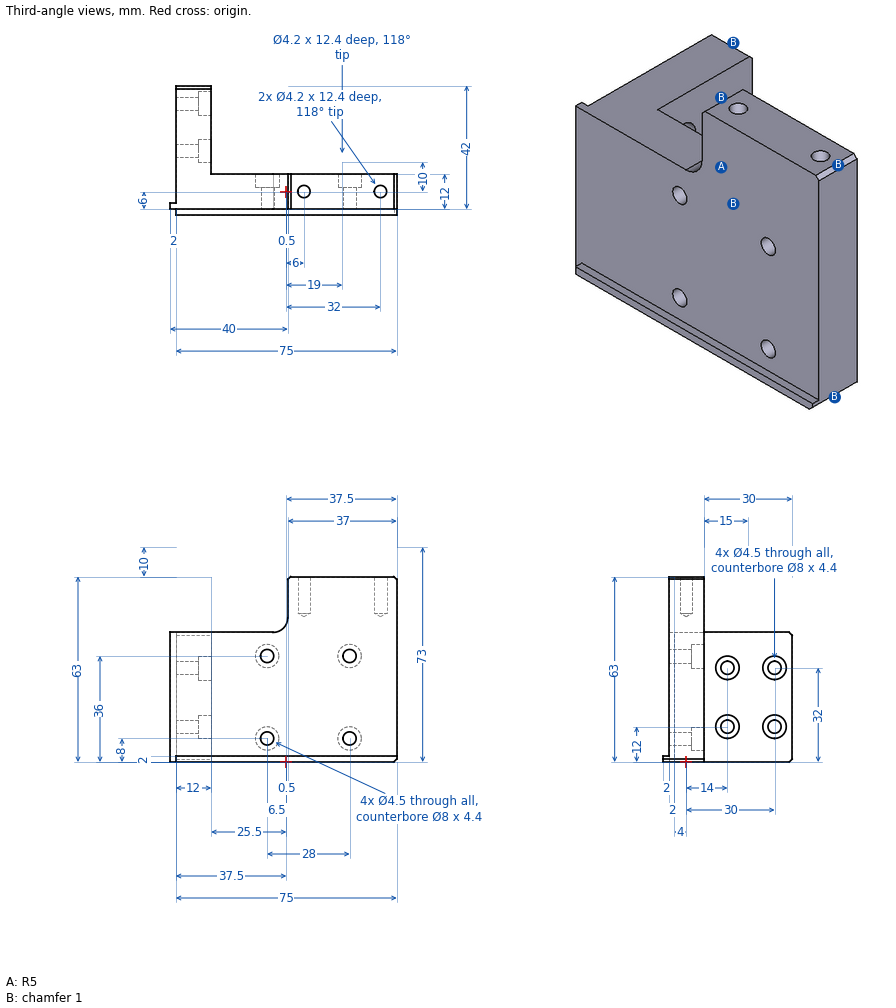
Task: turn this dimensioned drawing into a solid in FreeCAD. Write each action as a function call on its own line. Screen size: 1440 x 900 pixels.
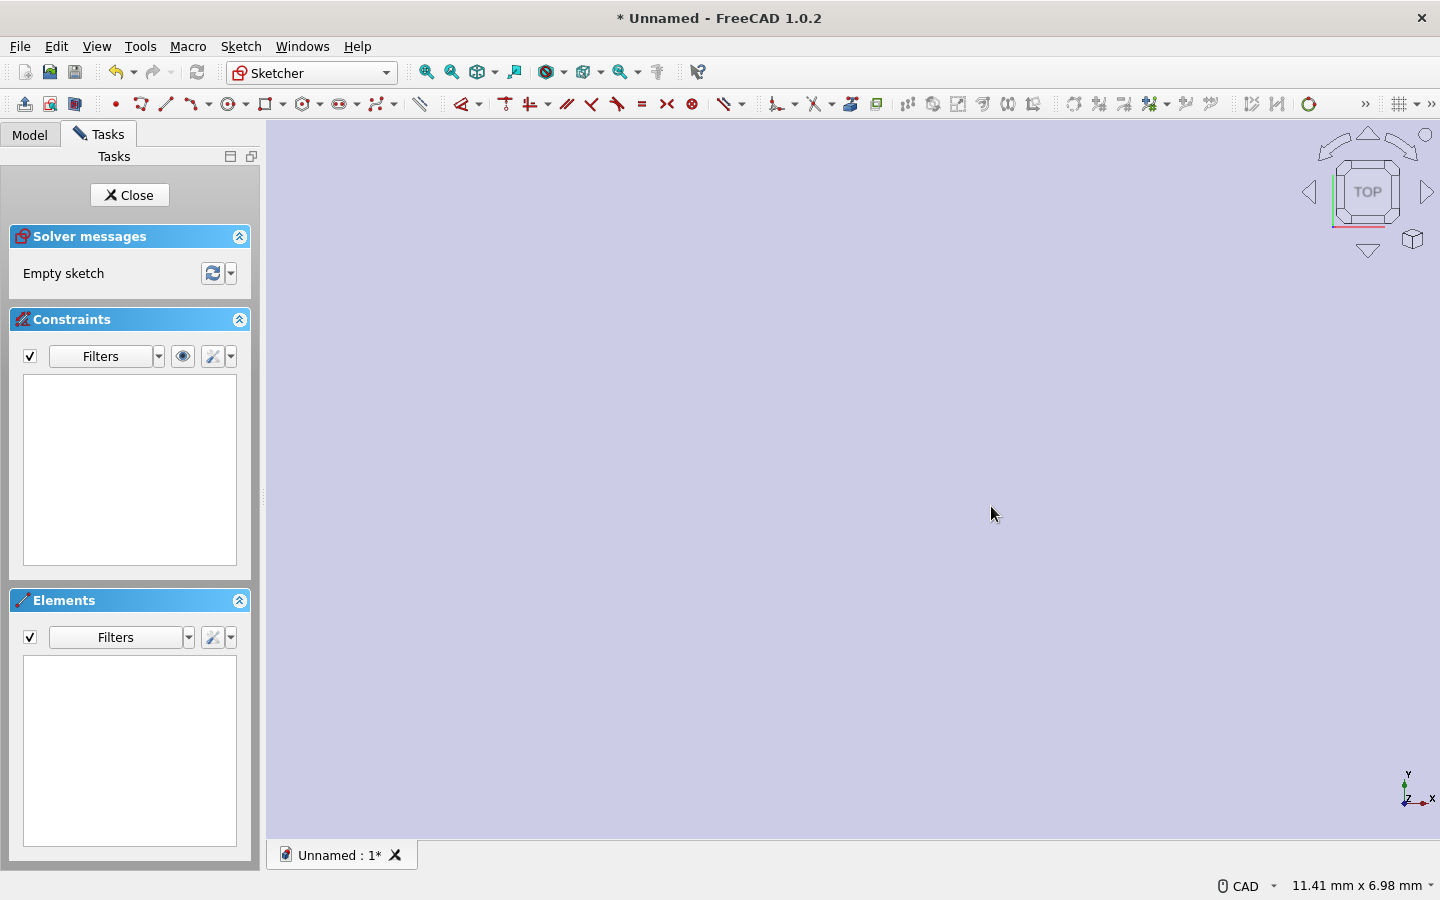
key(g)
key(c)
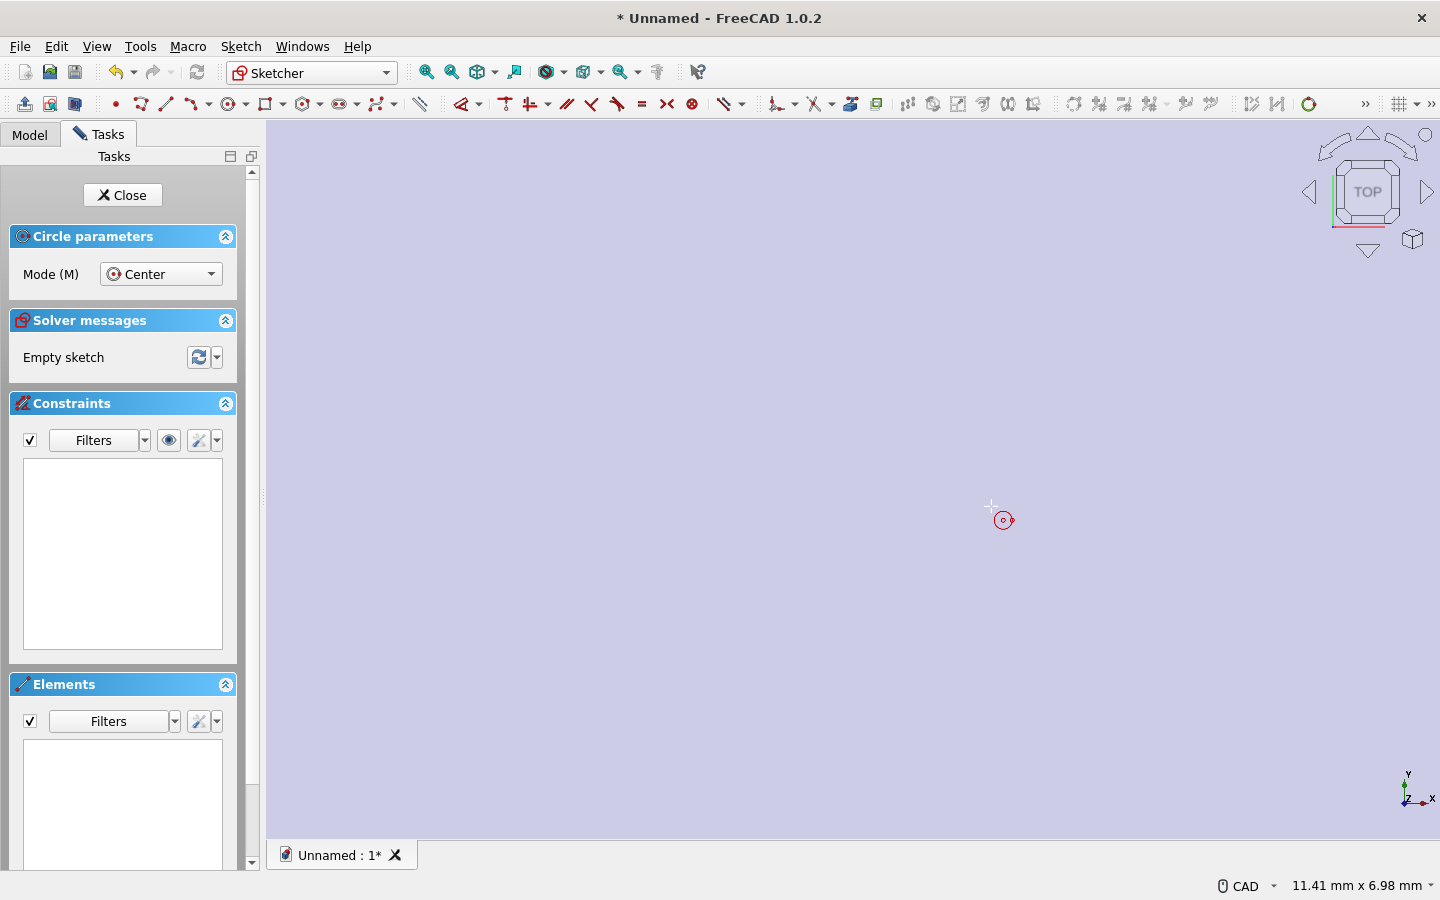
click(771, 474)
move(924, 321)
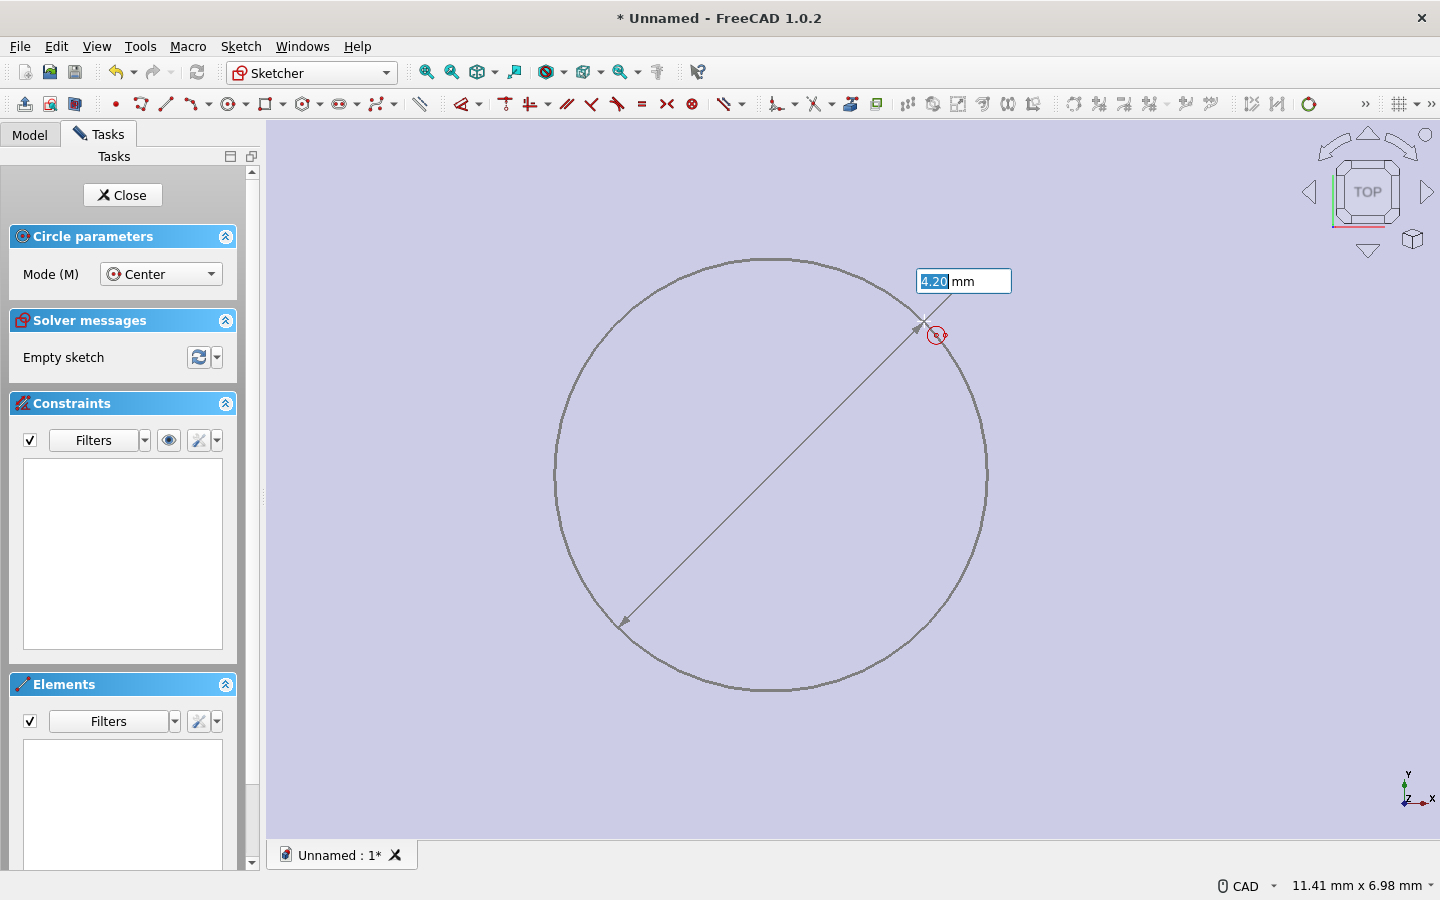
text(4.2)
key(Return)
key(Escape)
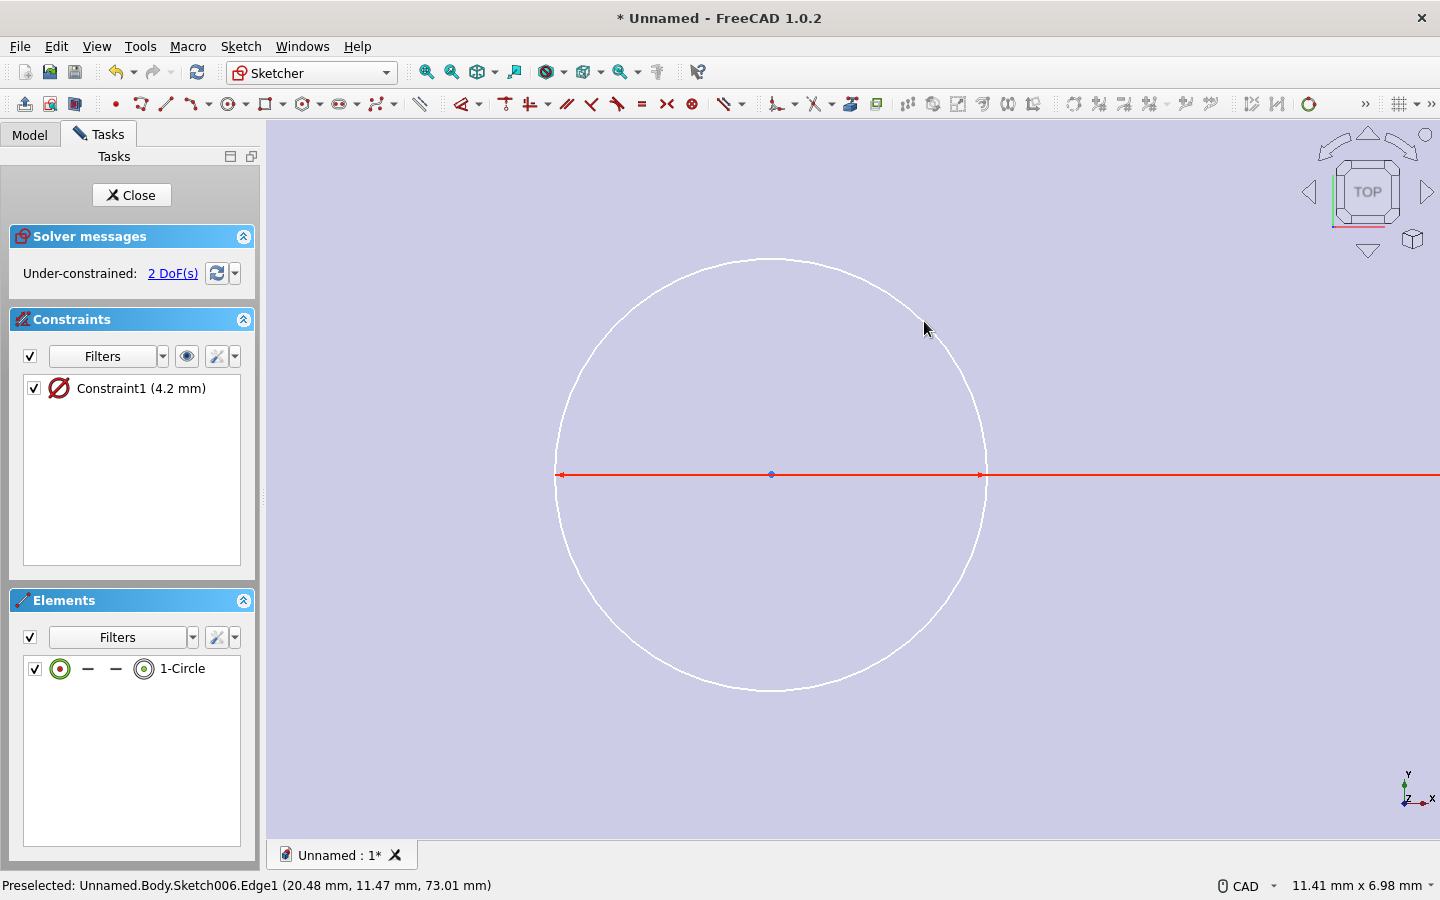
key(d)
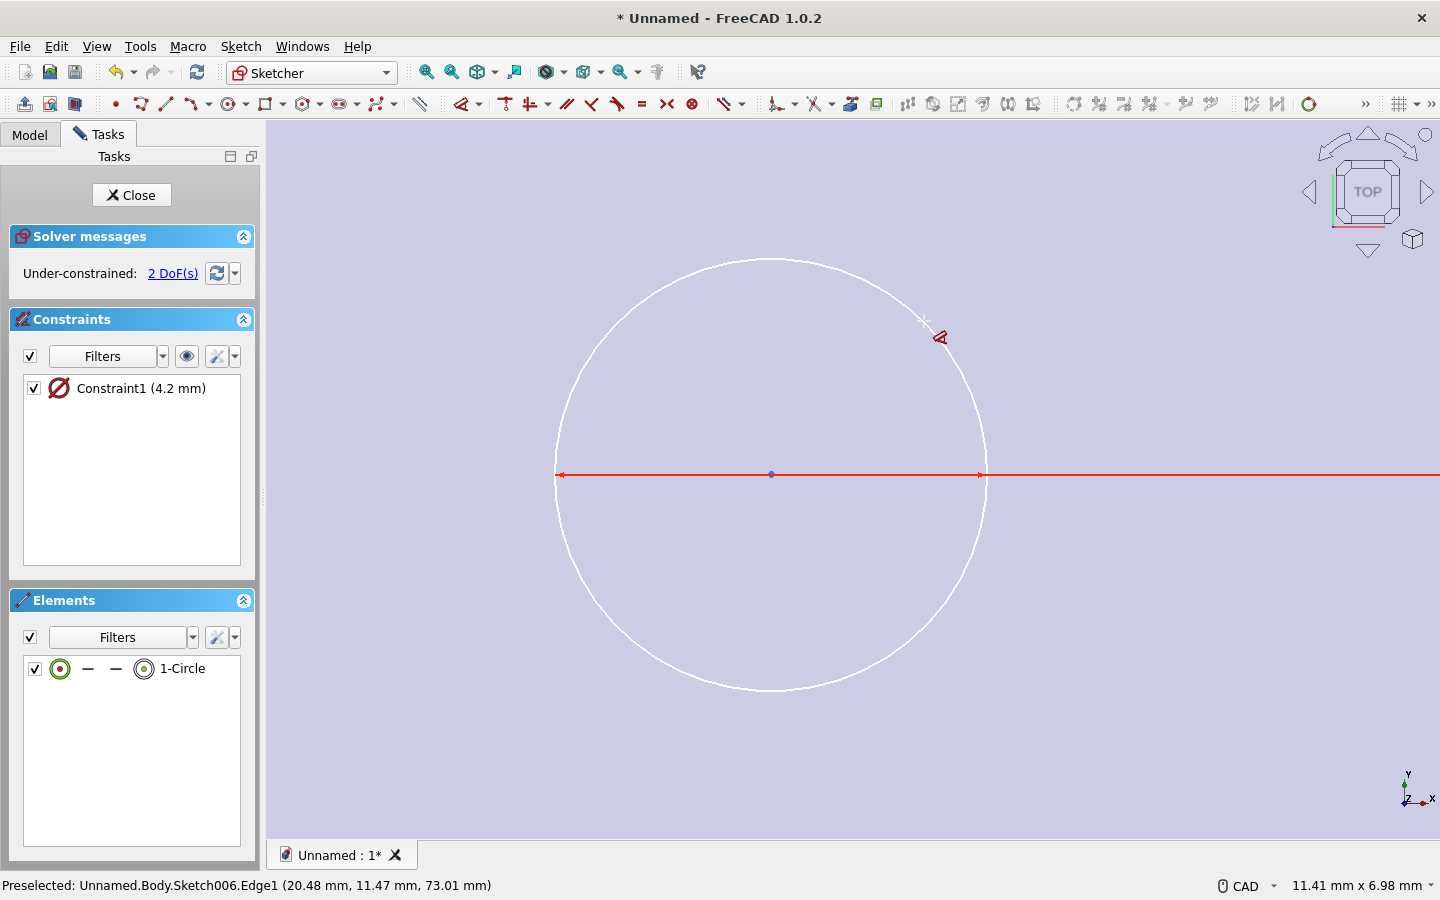
click(771, 475)
click(533, 441)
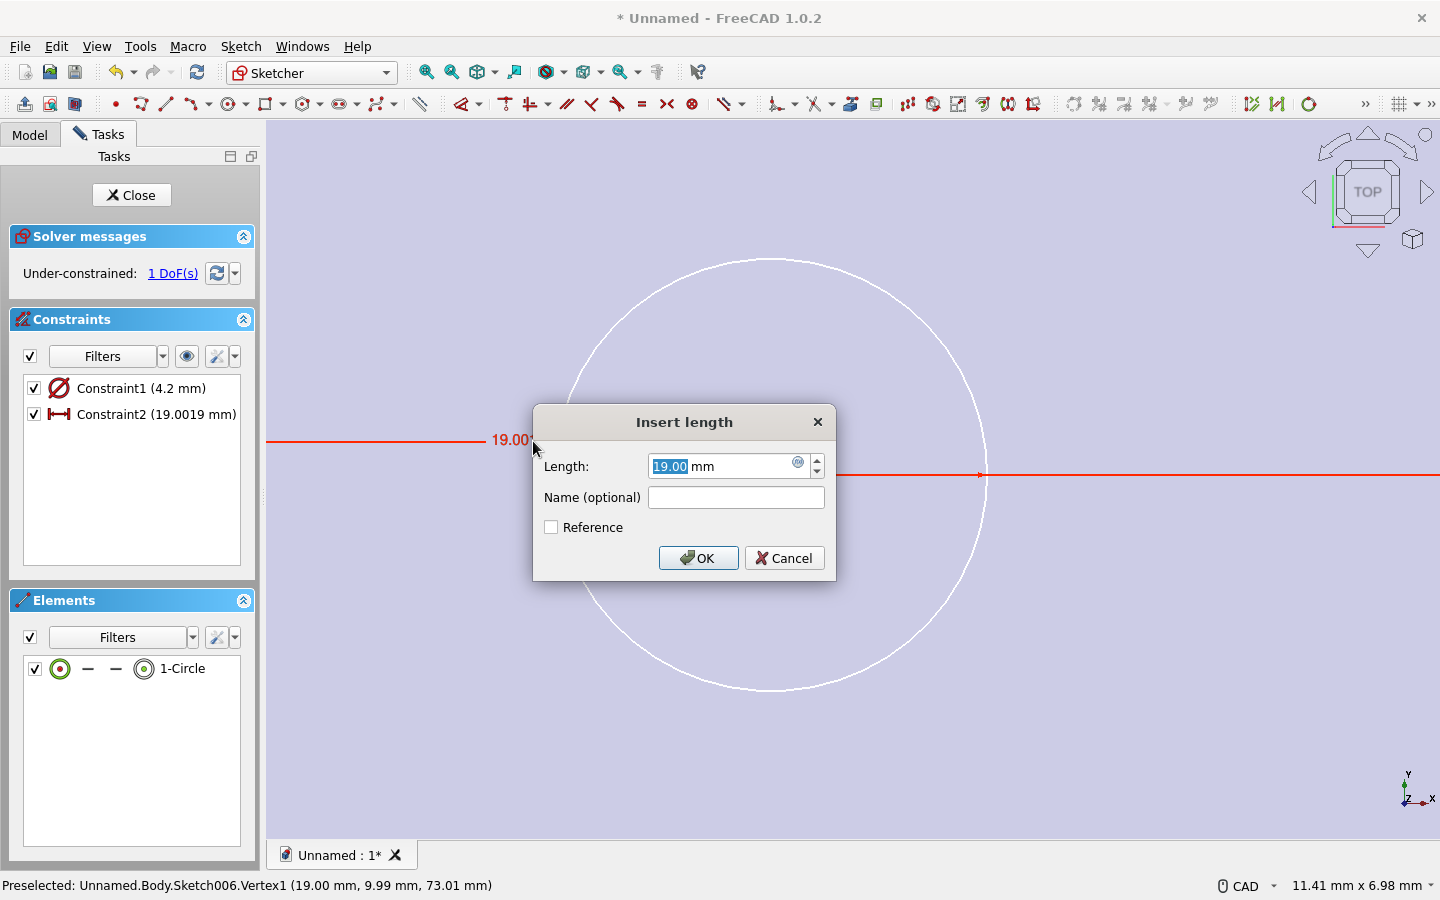
text(19)
key(Return)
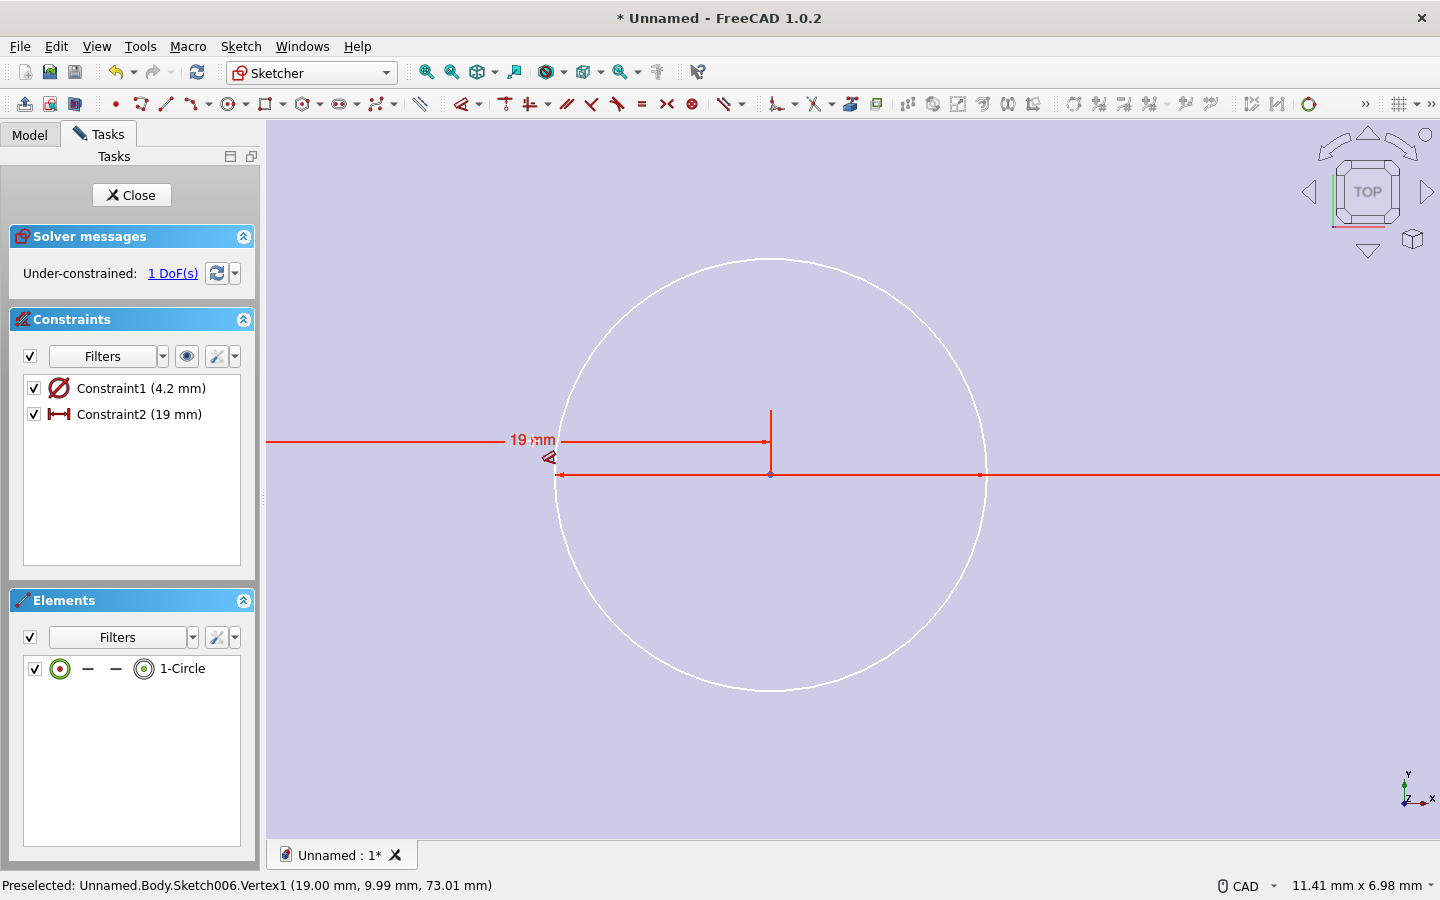
click(771, 475)
click(805, 643)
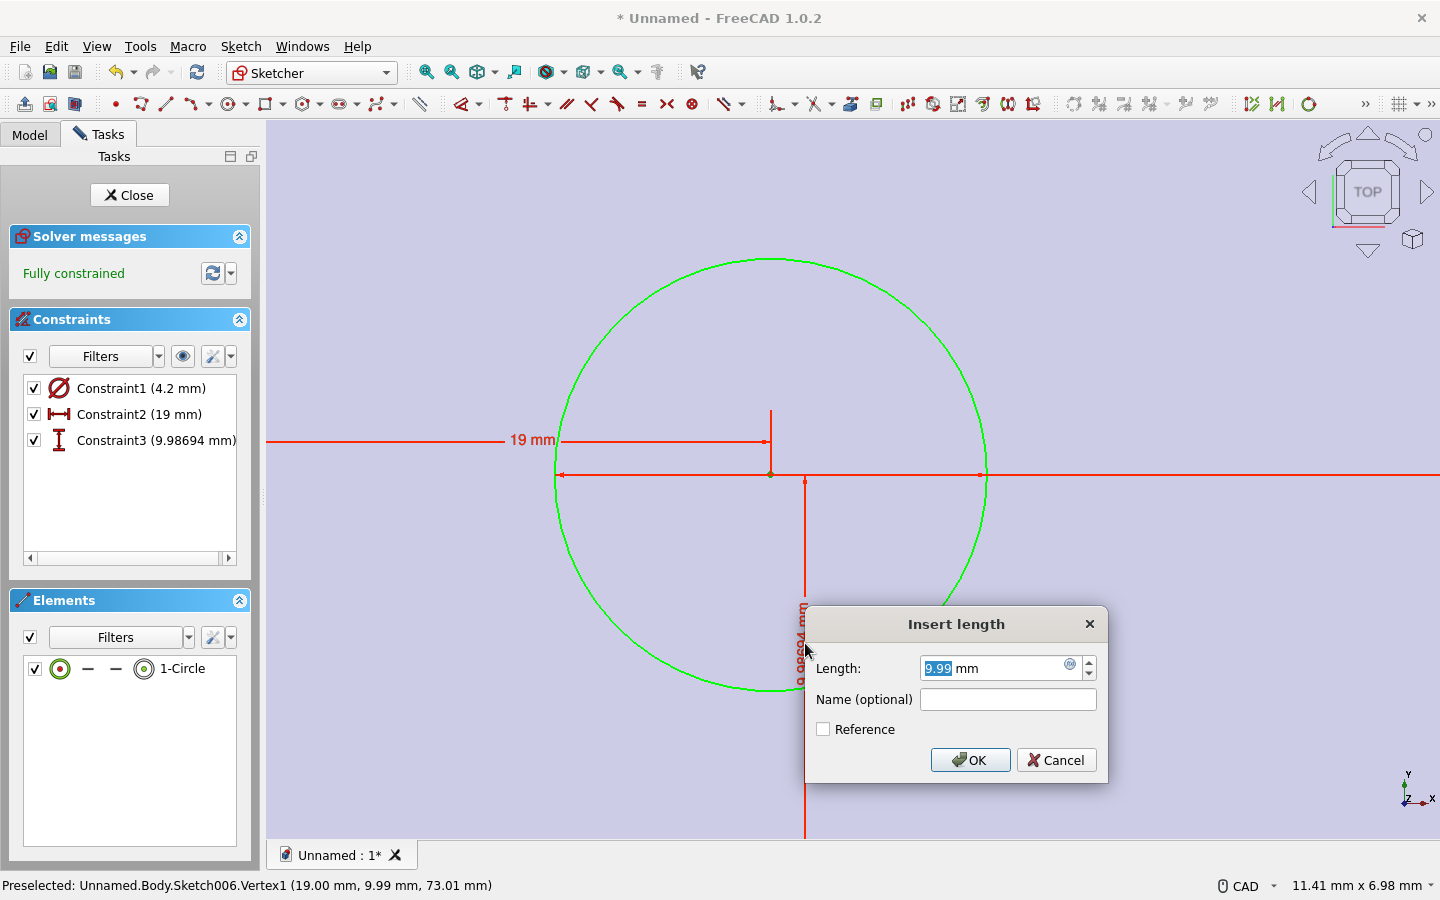
text(10)
key(Return)
key(Escape)